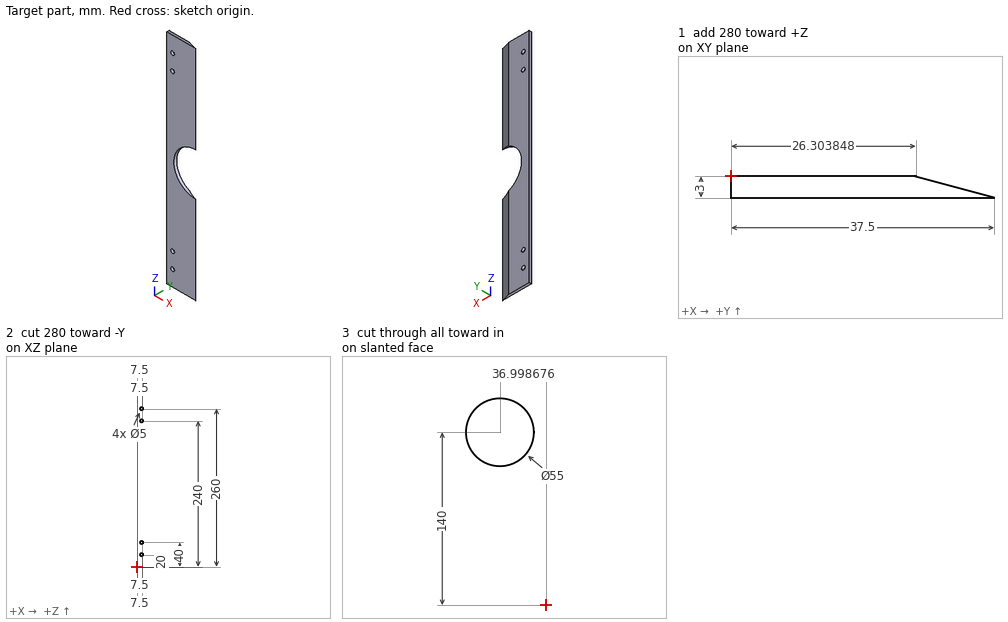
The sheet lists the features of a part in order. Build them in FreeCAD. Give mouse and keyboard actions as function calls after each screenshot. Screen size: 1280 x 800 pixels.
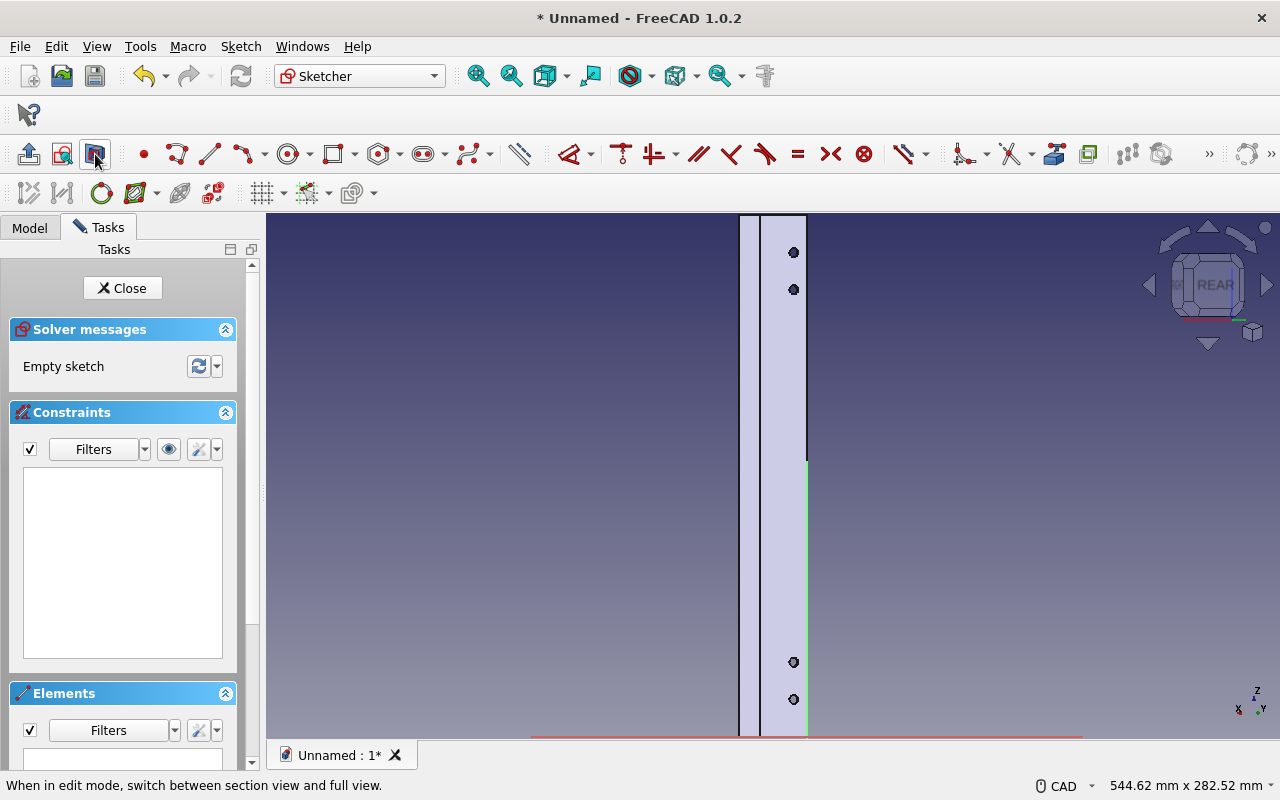
scroll(753, 476, up, 6)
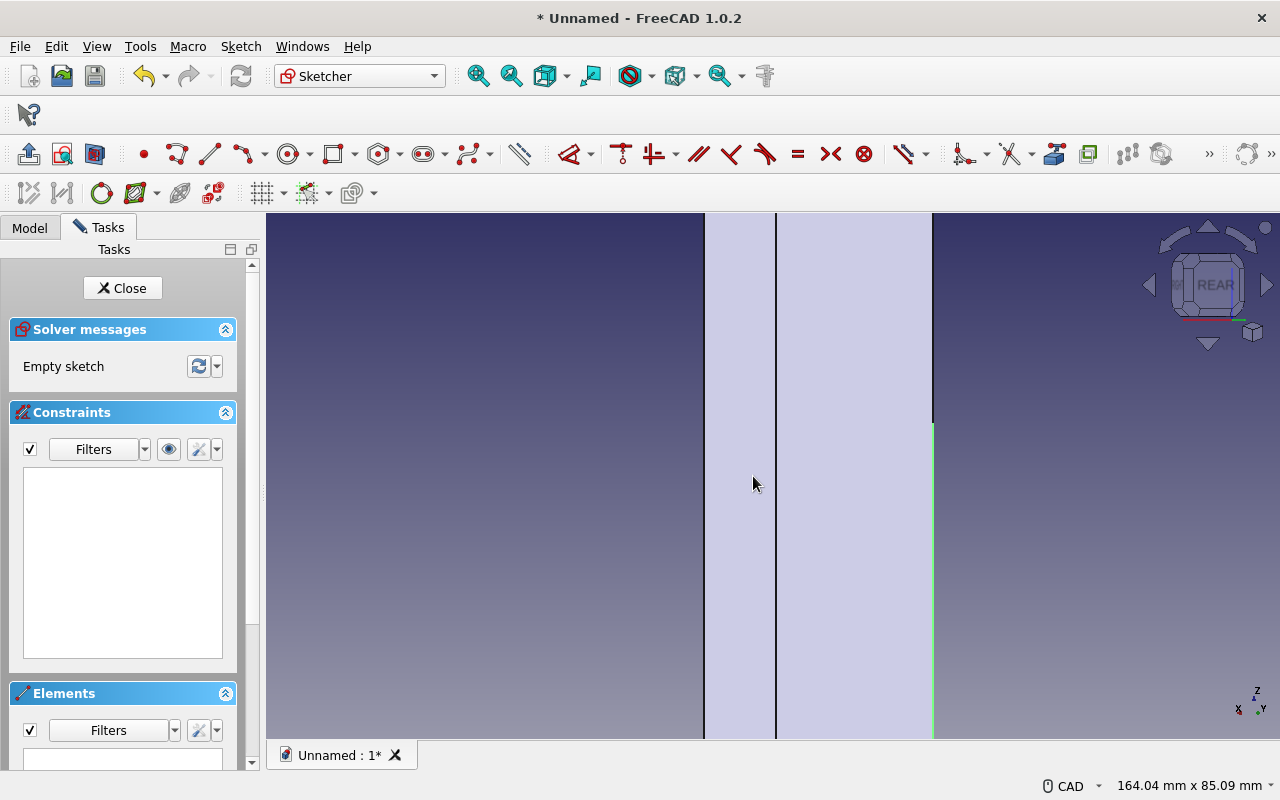
click(288, 154)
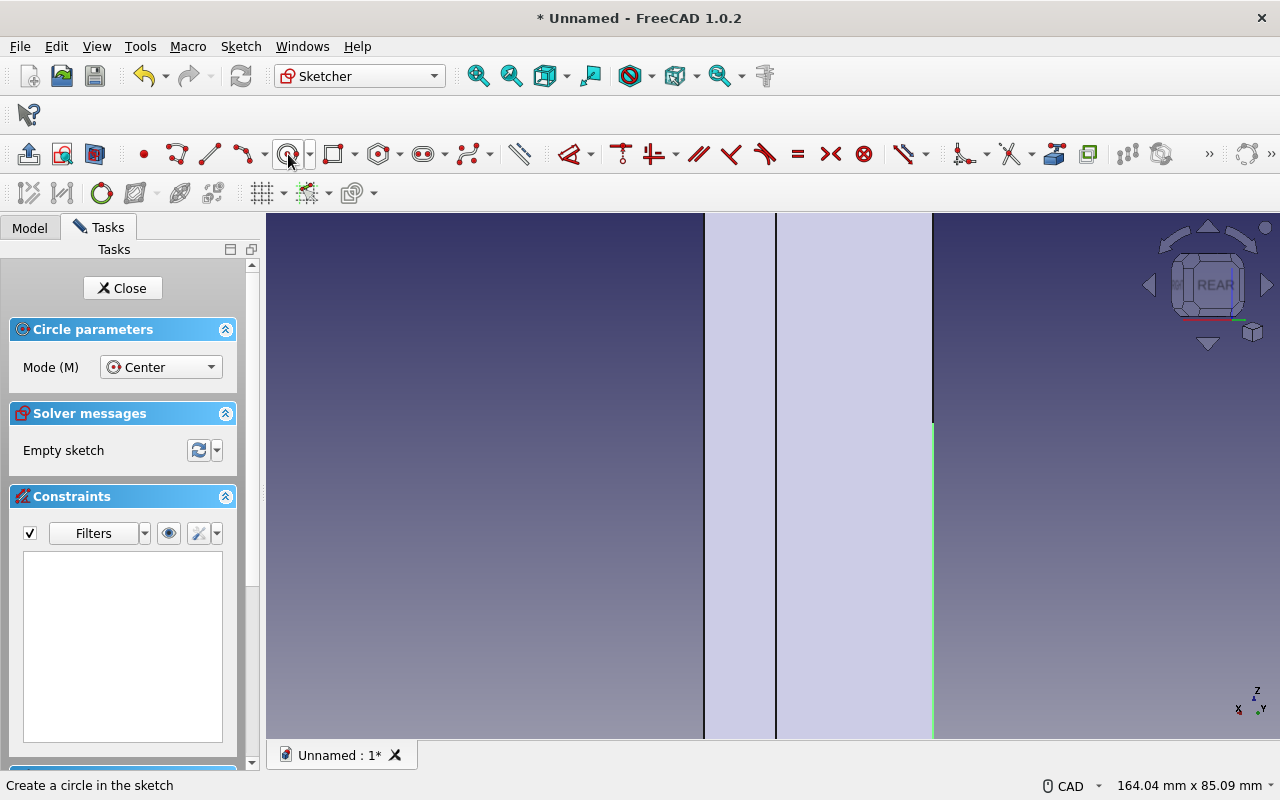
click(704, 475)
move(824, 355)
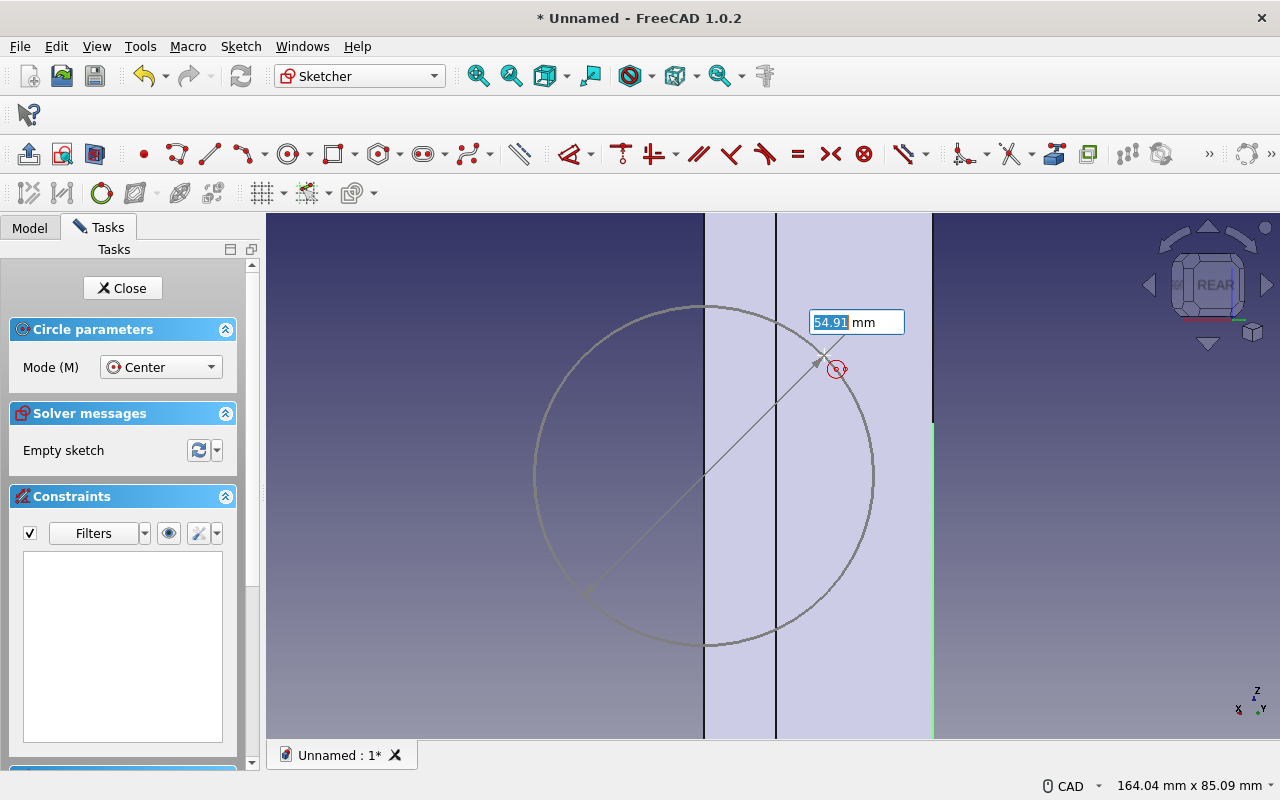
text(55)
key(Return)
key(Escape)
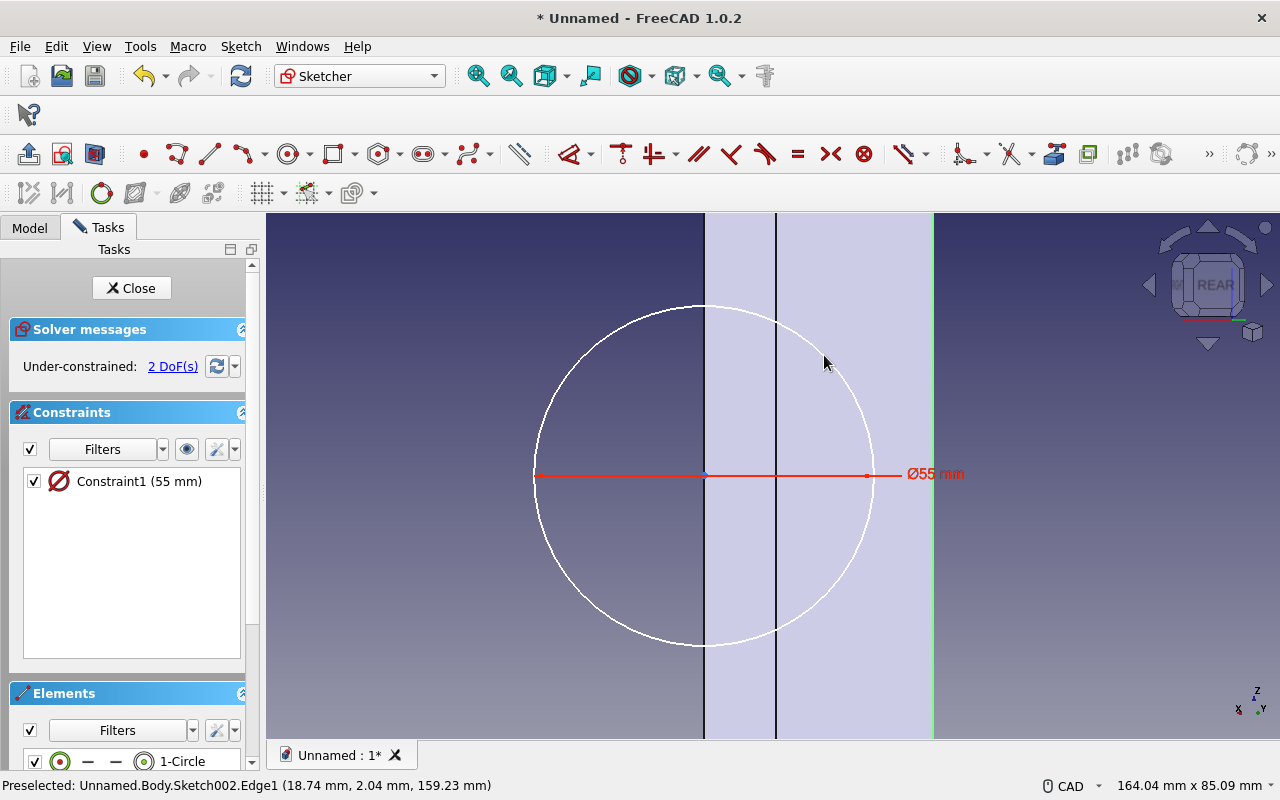
click(568, 154)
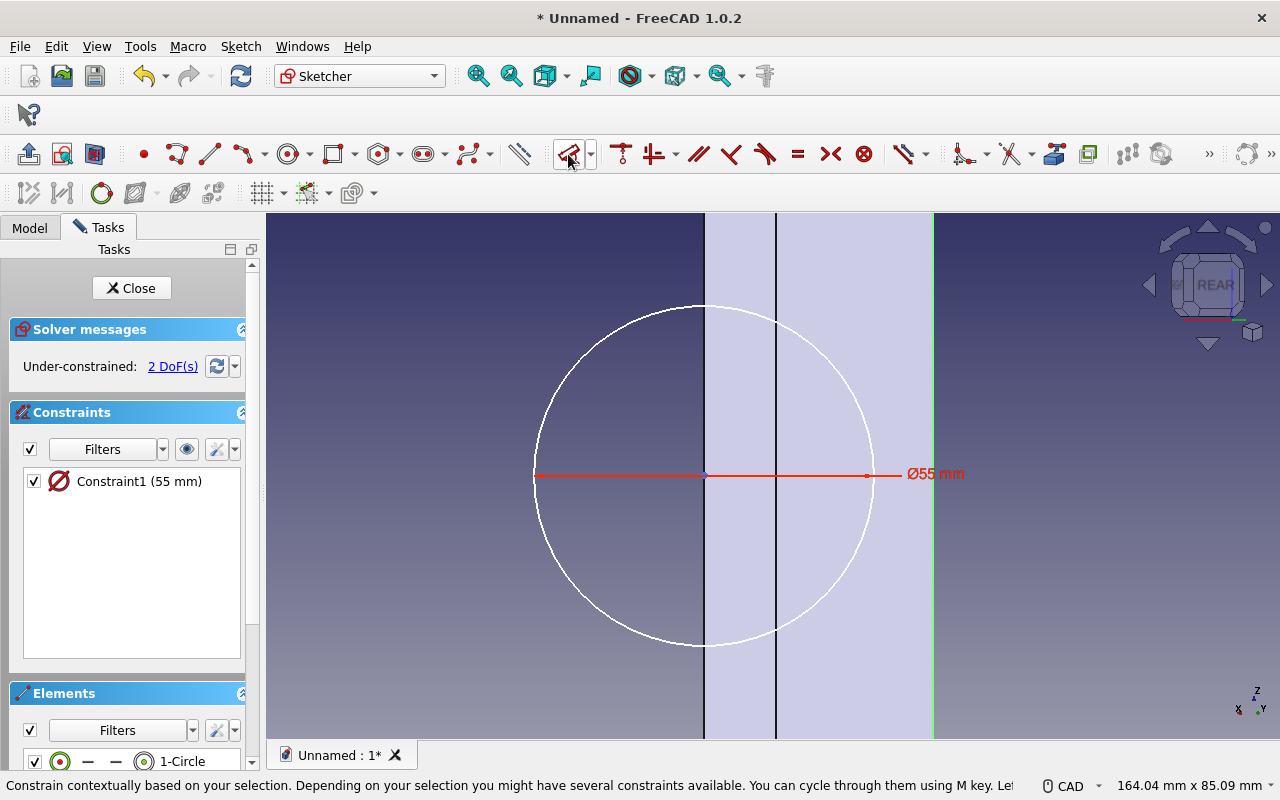
click(704, 476)
click(967, 593)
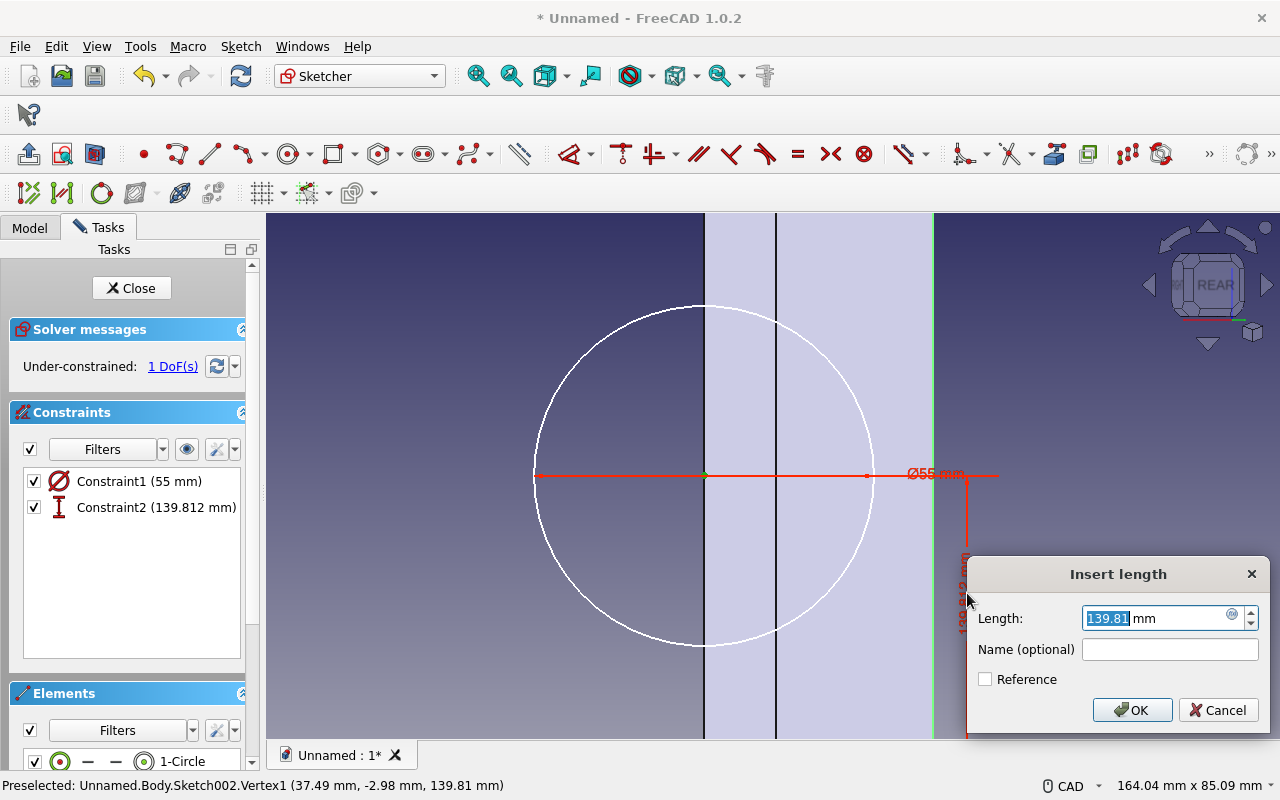
text(140)
key(Return)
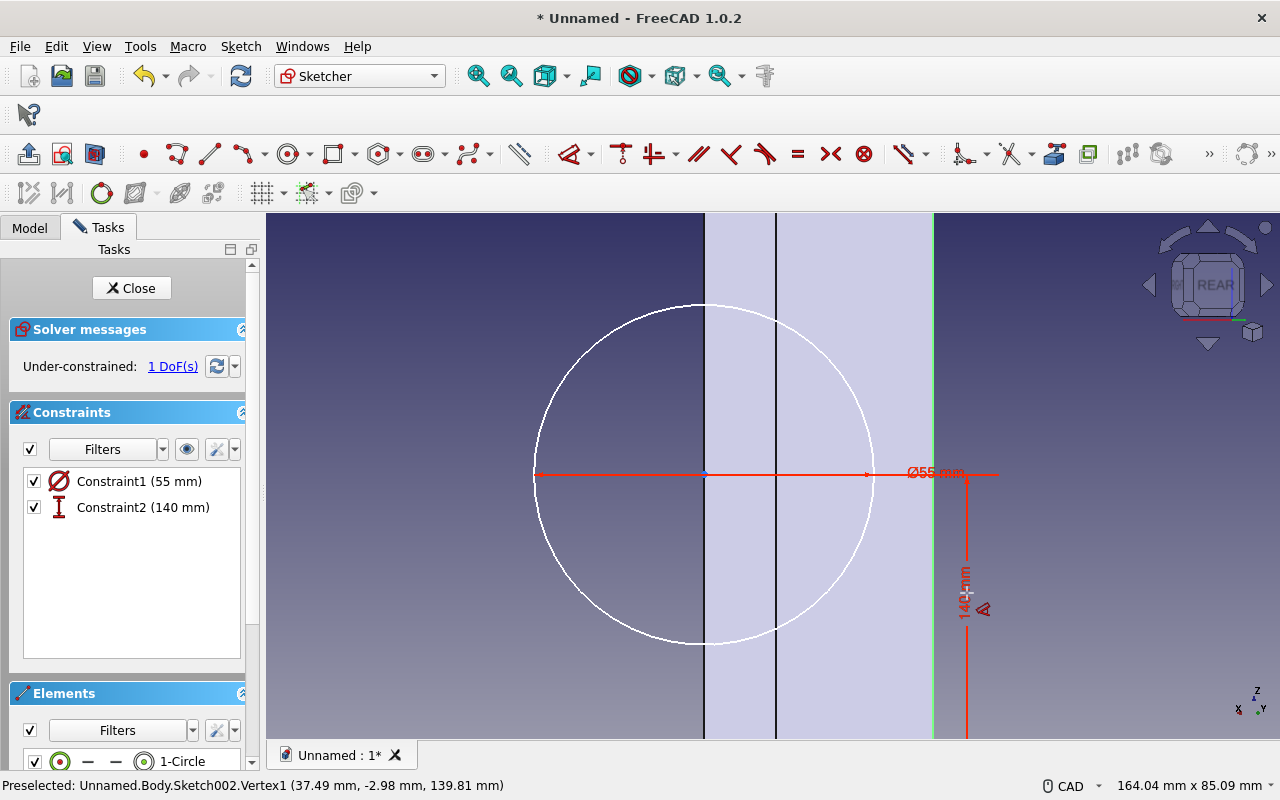
click(704, 475)
click(818, 441)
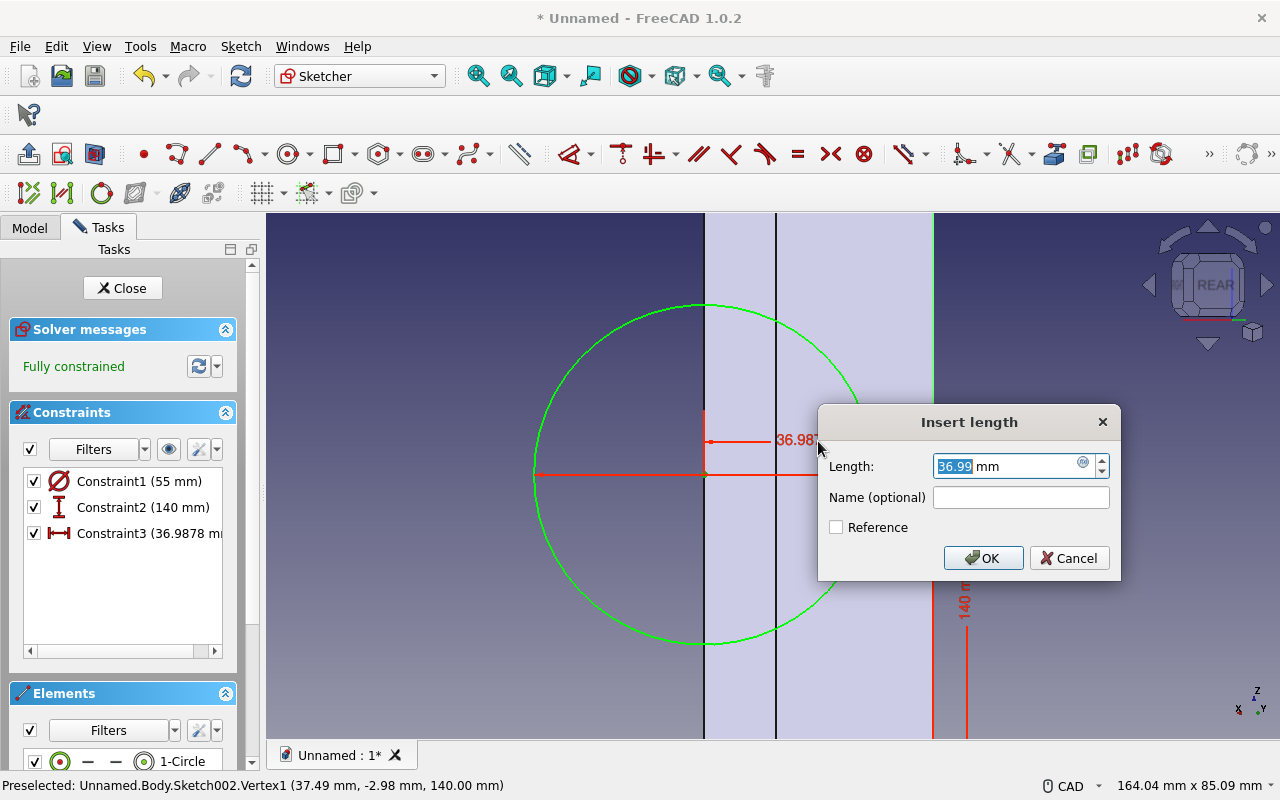
text(36.998676)
key(Return)
key(Escape)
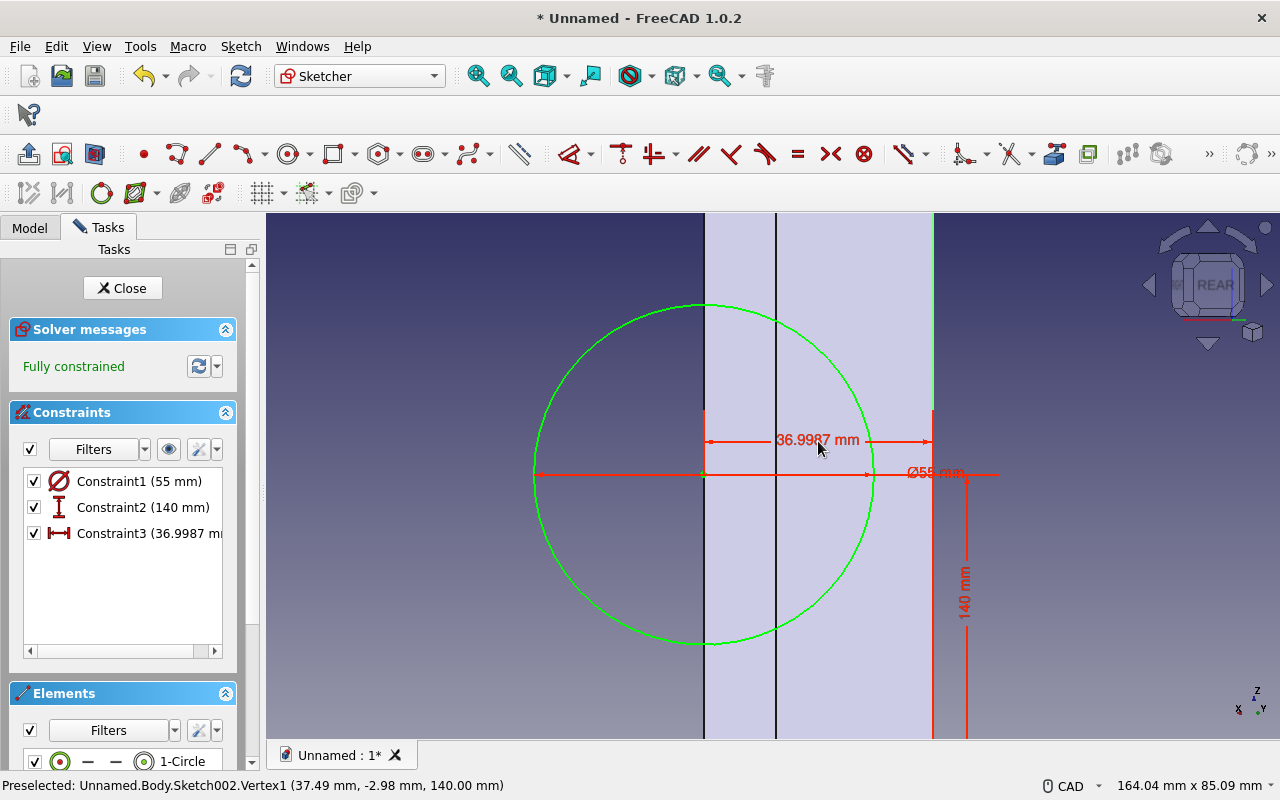
click(123, 288)